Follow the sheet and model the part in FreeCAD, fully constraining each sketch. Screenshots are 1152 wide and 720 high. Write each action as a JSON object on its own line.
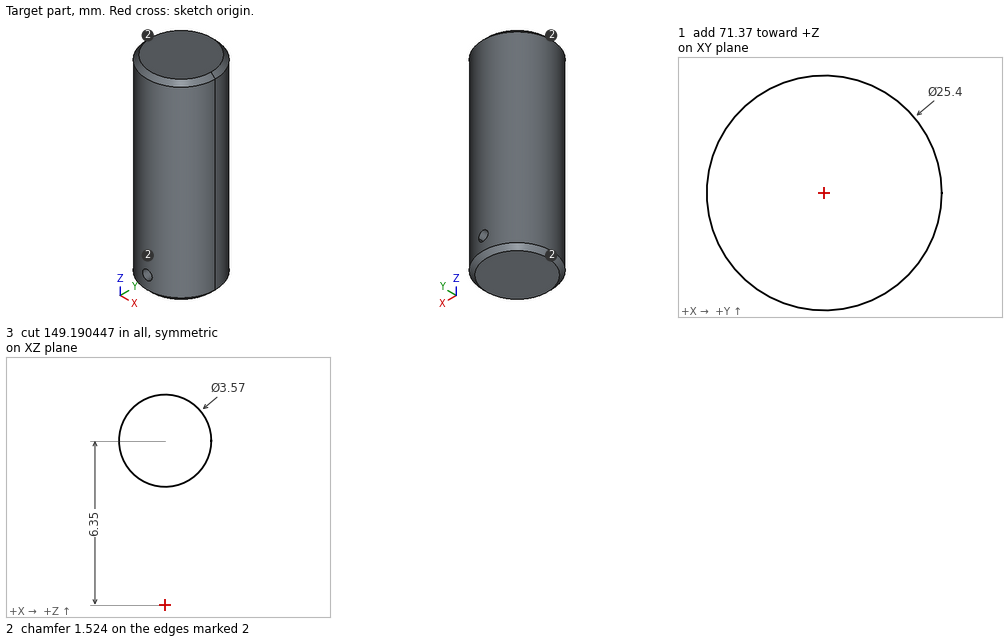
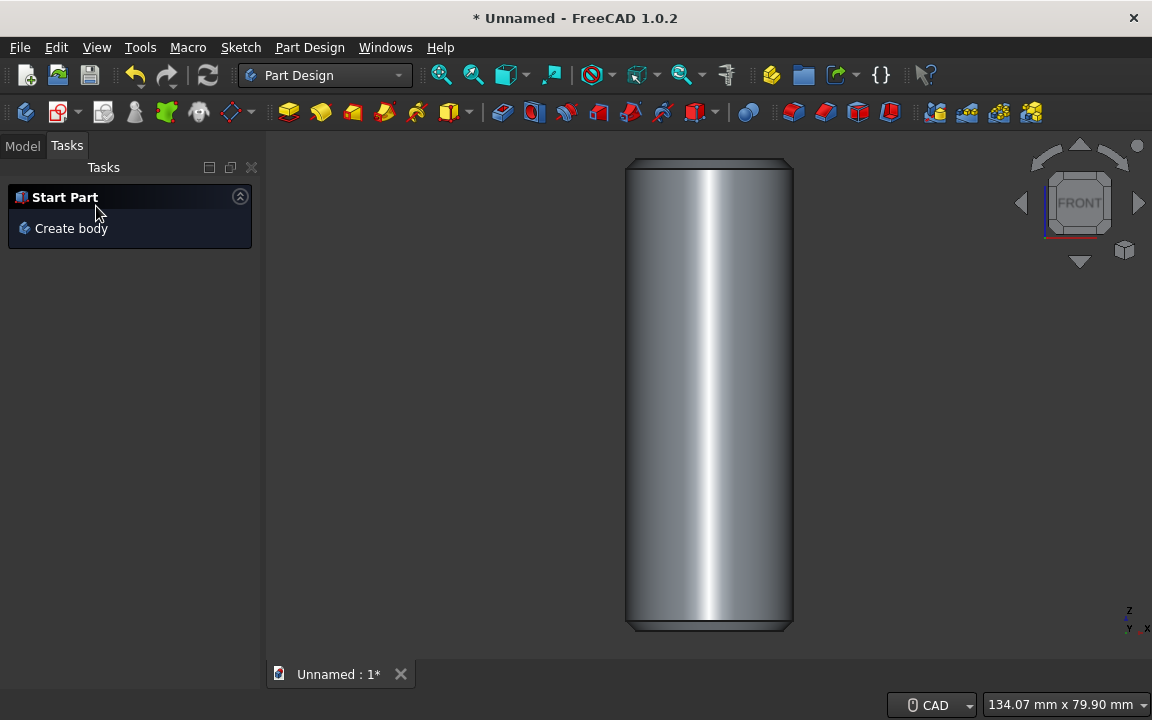
{"action": "left_click", "coordinate": [58, 112]}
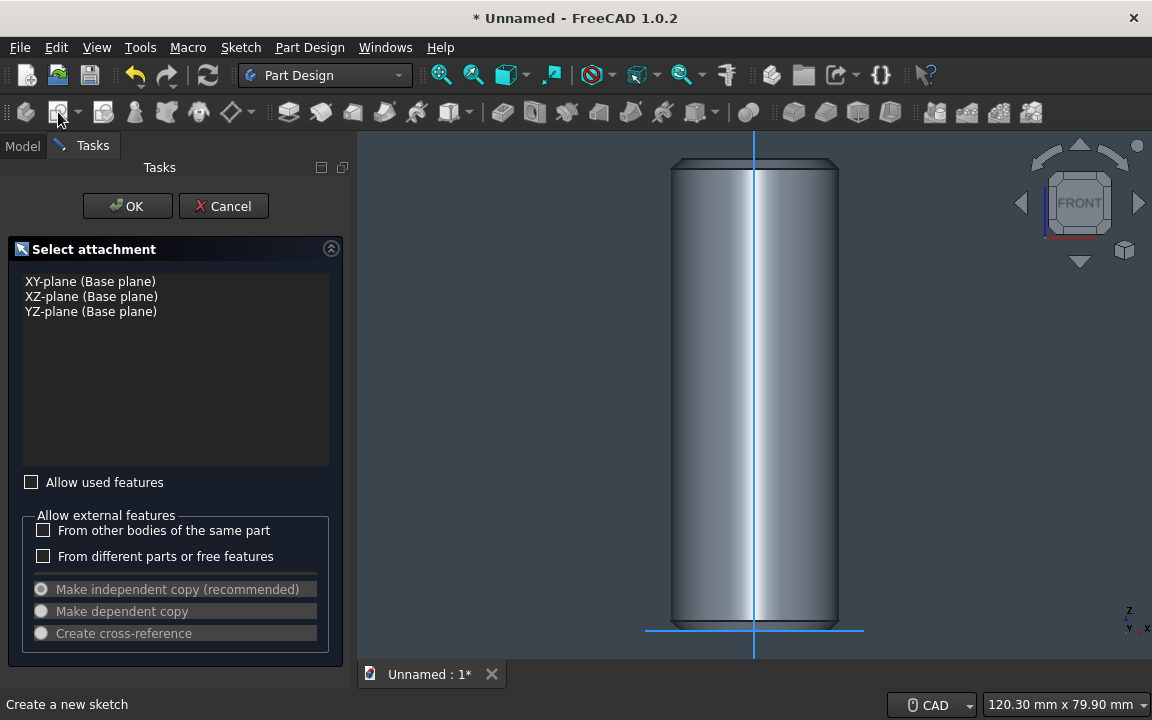
{"action": "left_click", "coordinate": [82, 296]}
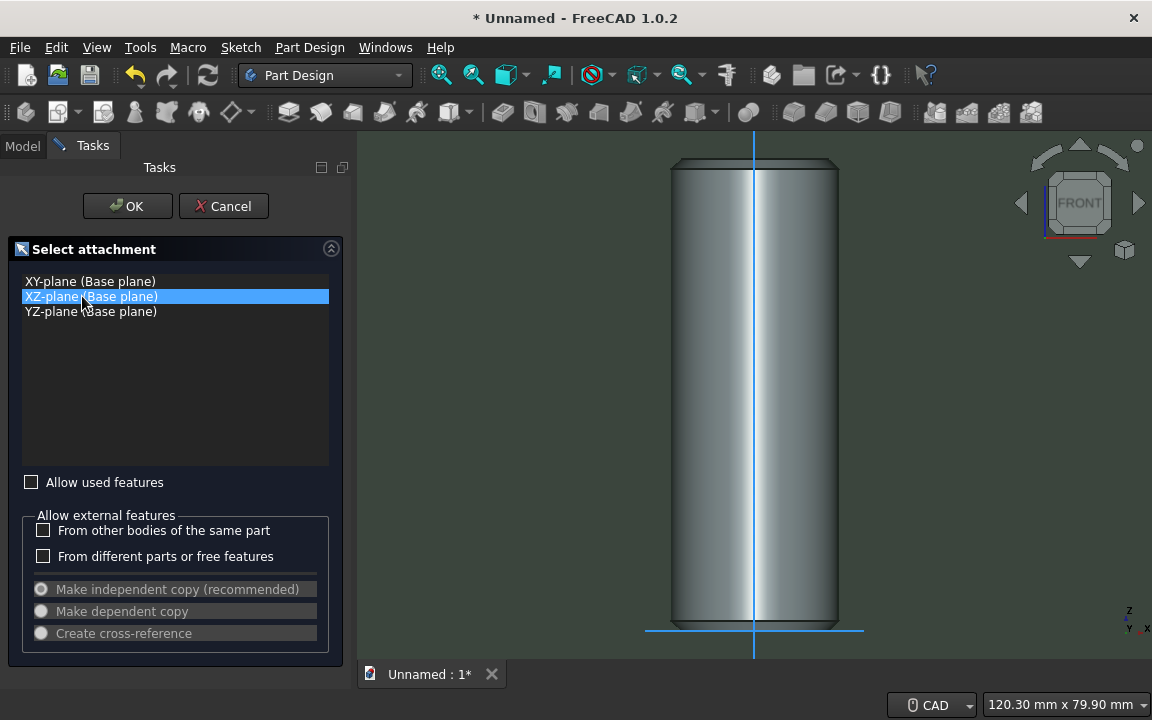
{"action": "left_click", "coordinate": [128, 206]}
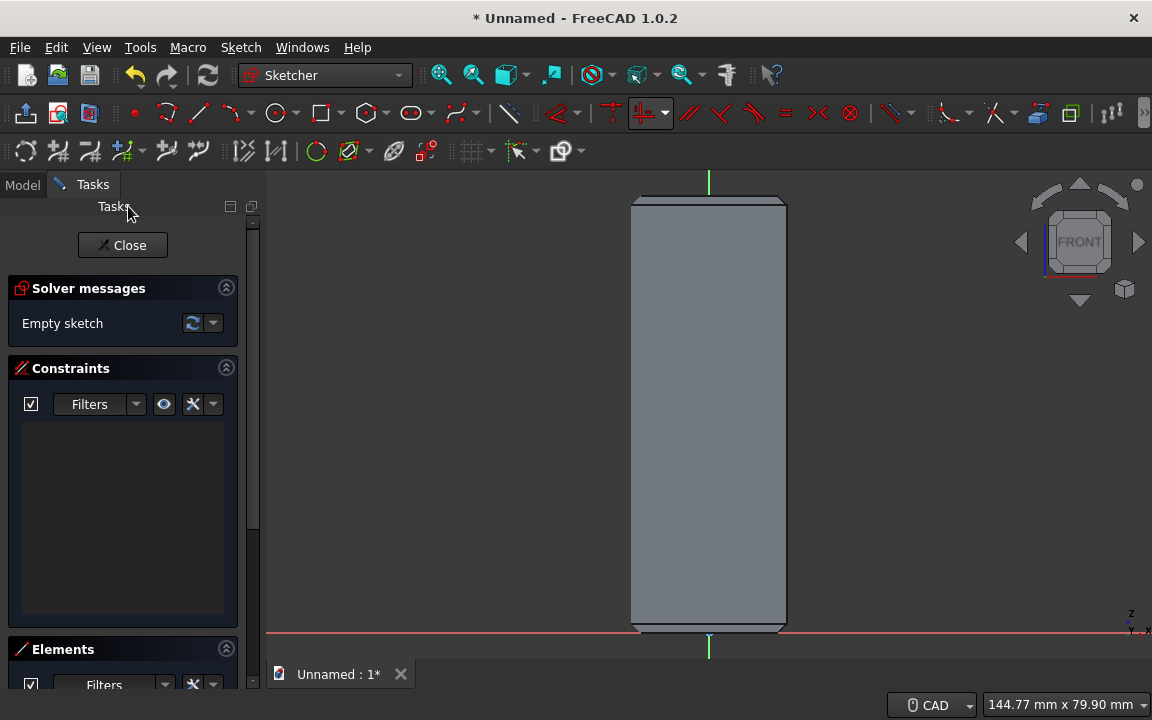
{"action": "left_click", "coordinate": [90, 114]}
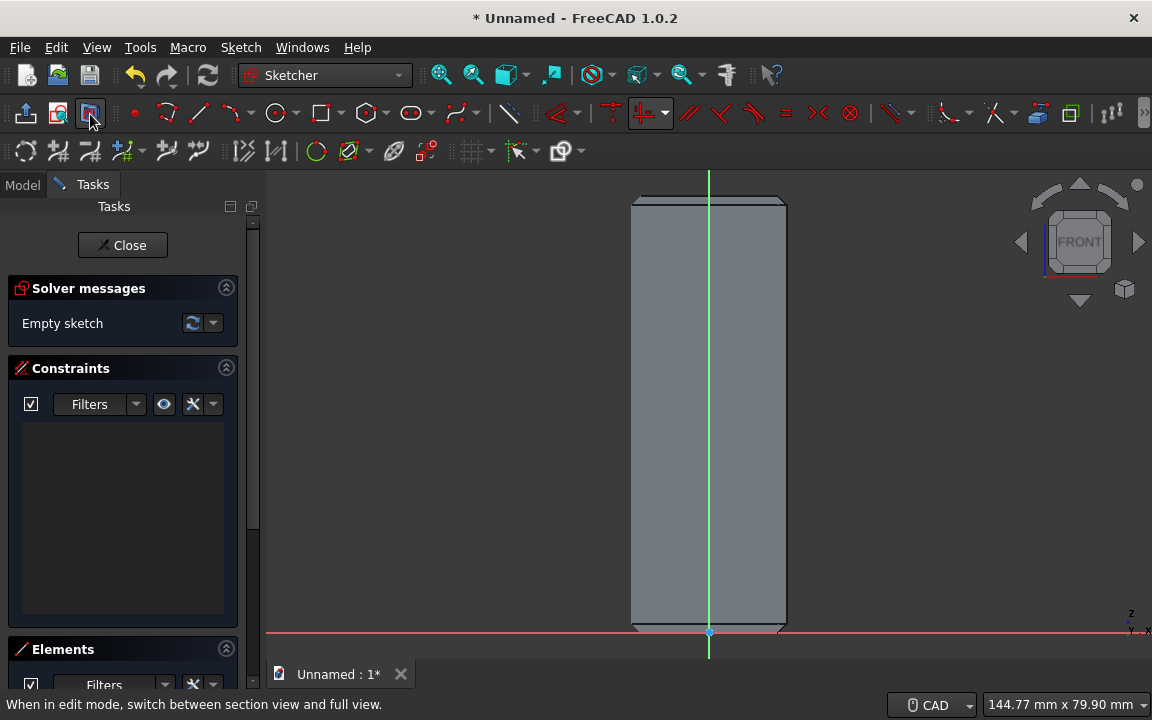
{"action": "scroll", "coordinate": [640, 414], "scroll_direction": "down", "scroll_amount": 5}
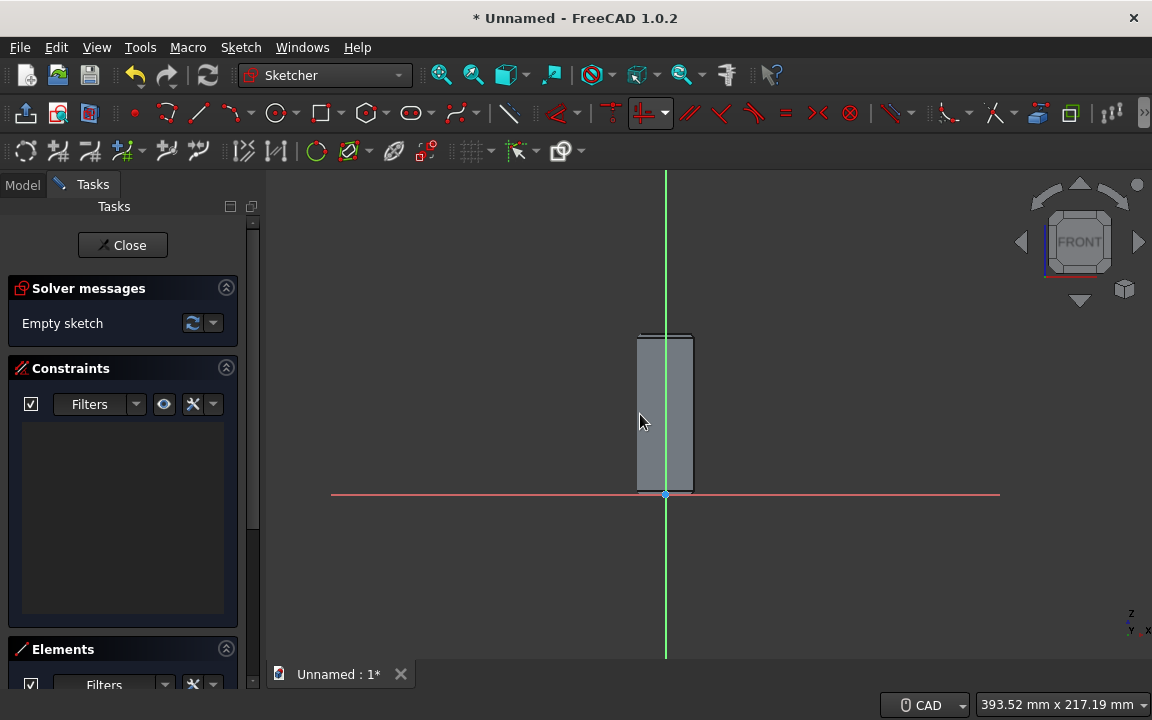
{"action": "scroll", "coordinate": [667, 490], "scroll_direction": "up", "scroll_amount": 14}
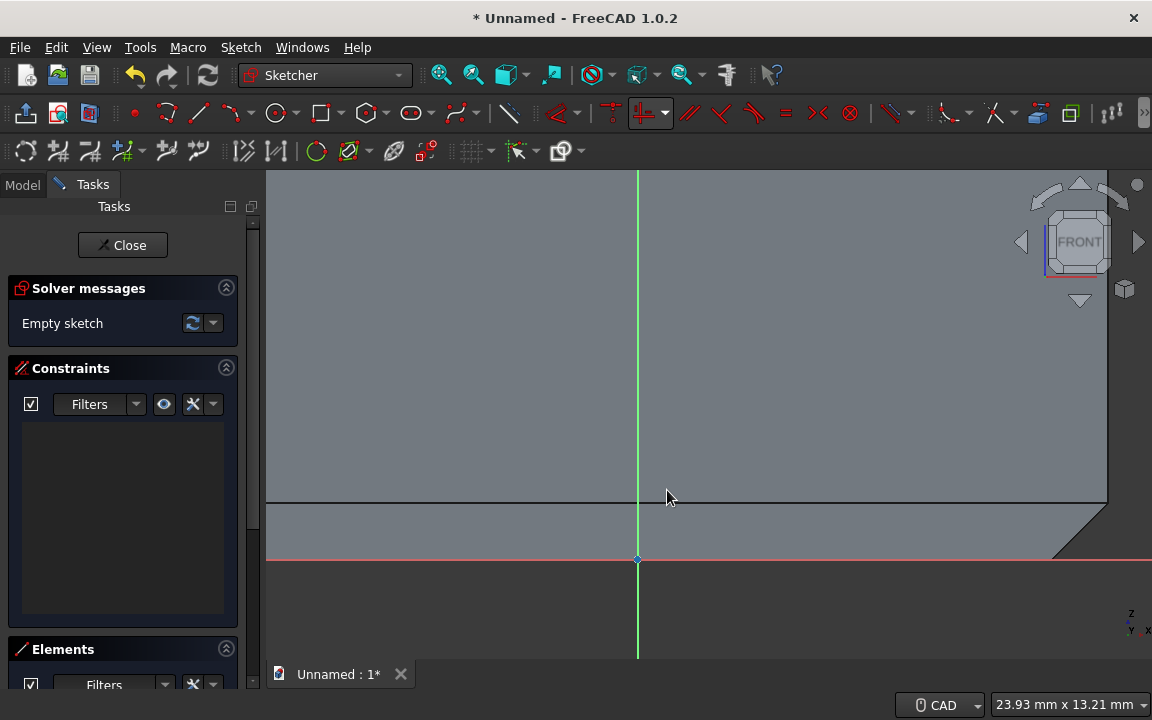
{"action": "left_click", "coordinate": [276, 114]}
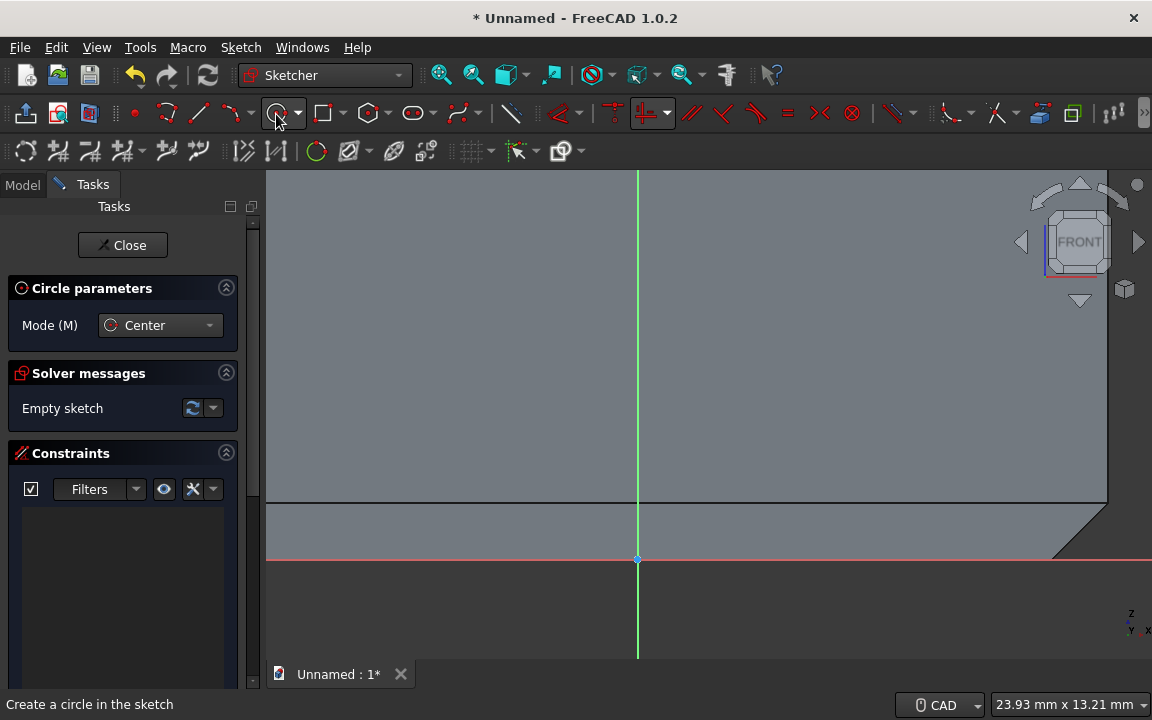
{"action": "left_click", "coordinate": [638, 324]}
{"action": "left_click", "coordinate": [685, 278]}
{"action": "key", "text": "Escape"}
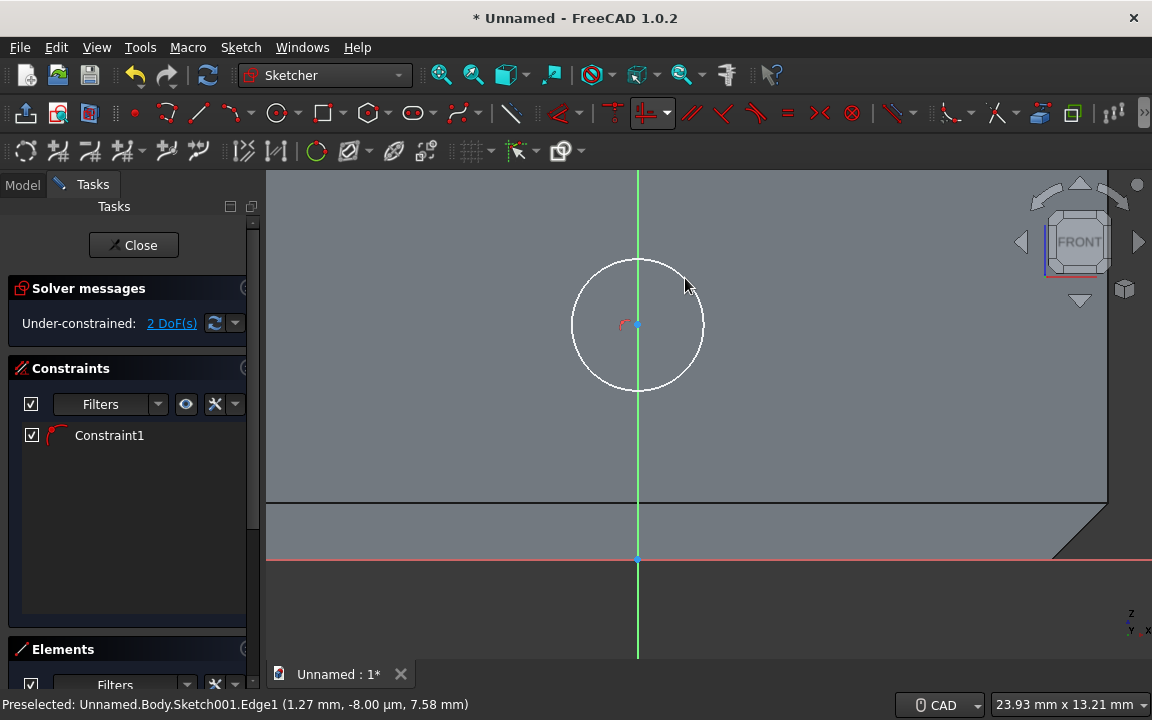
{"action": "left_click", "coordinate": [558, 114]}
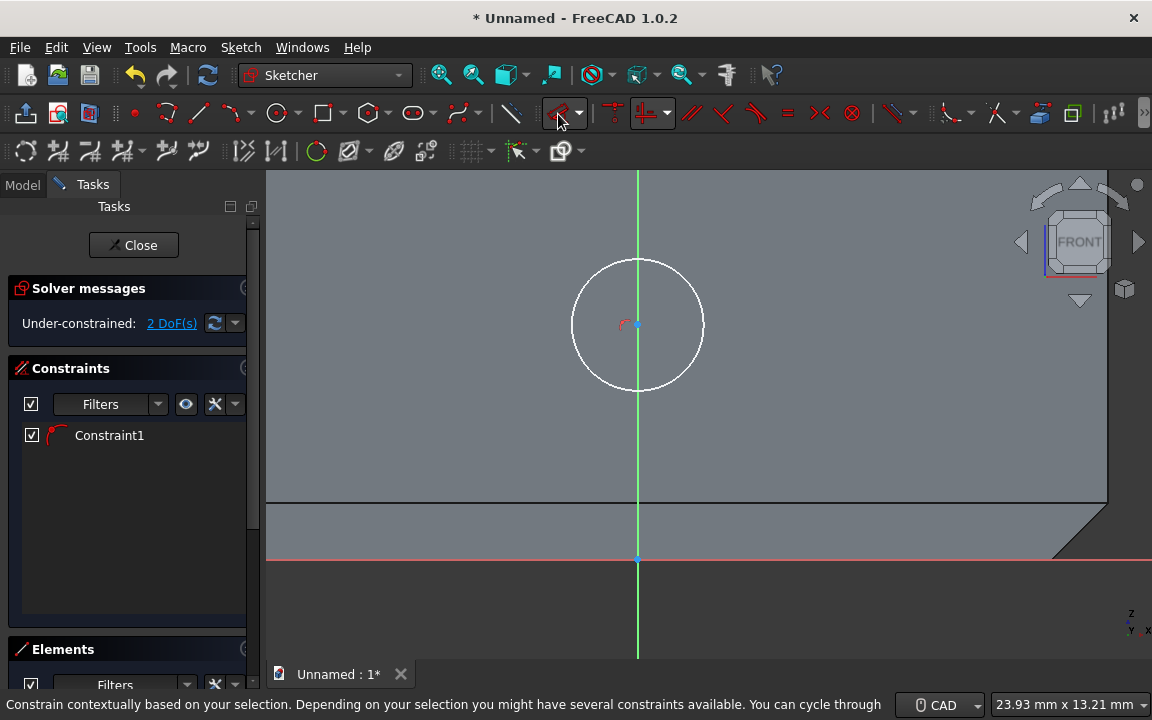
{"action": "left_click", "coordinate": [684, 278]}
{"action": "left_click", "coordinate": [706, 255]}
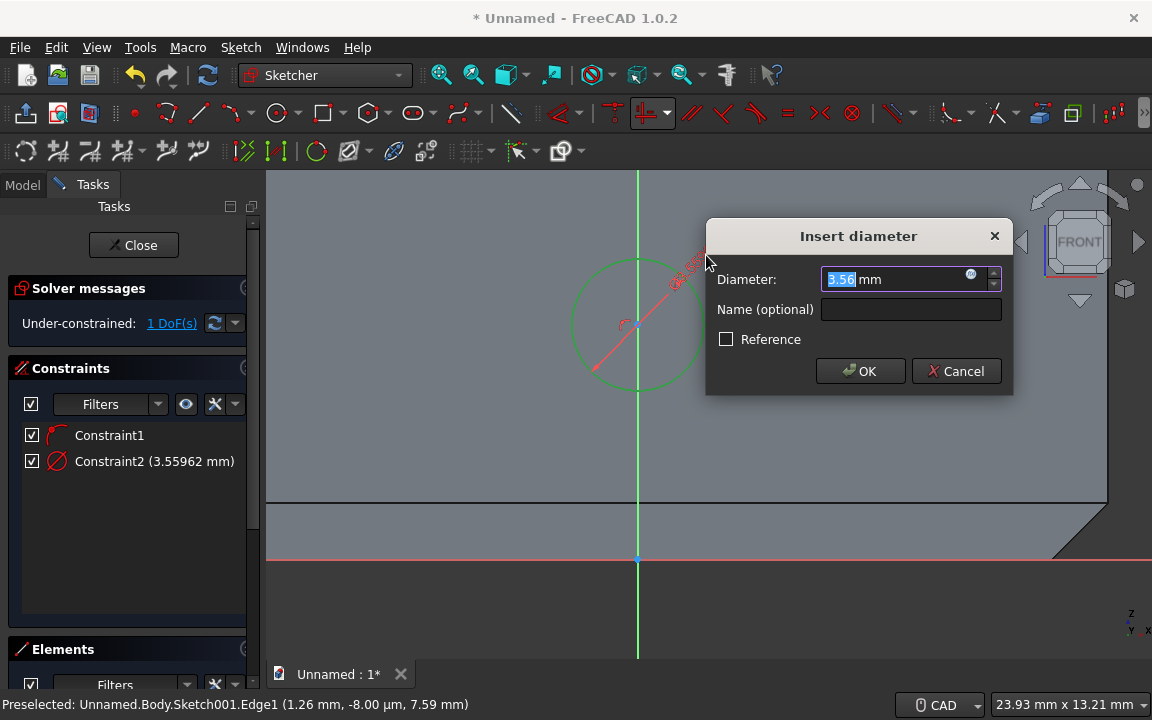
{"action": "type", "text": "3.57"}
{"action": "key", "text": "Return"}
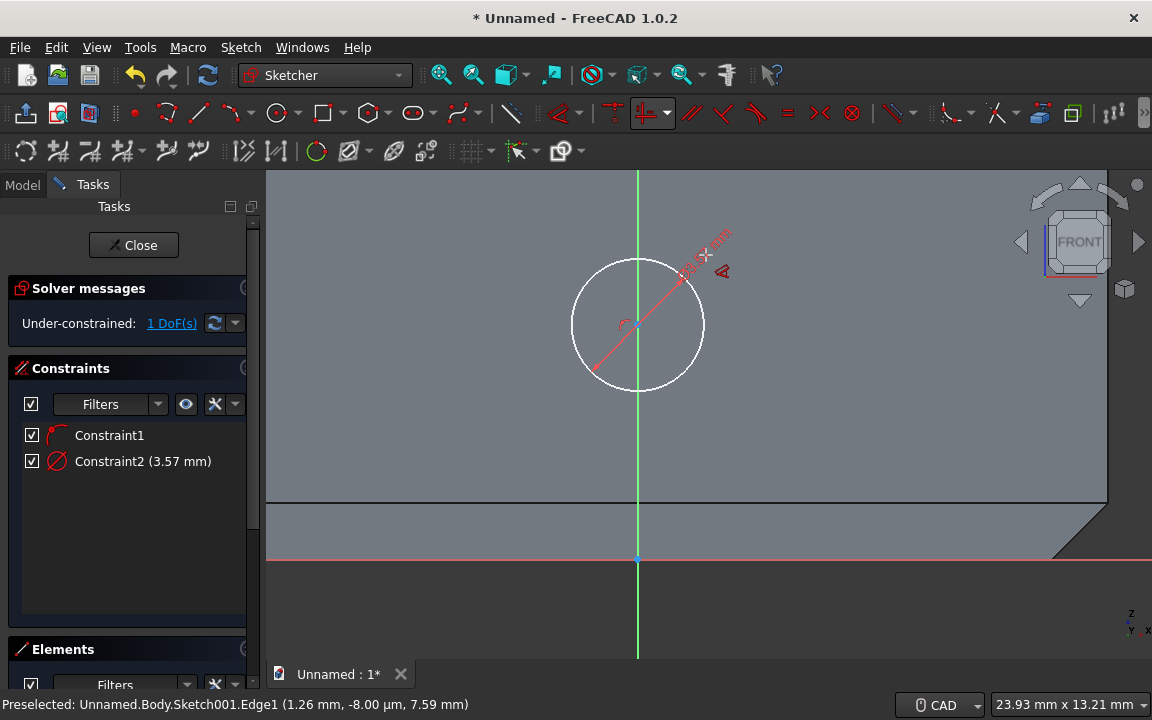
{"action": "left_click", "coordinate": [638, 325]}
{"action": "left_click", "coordinate": [672, 442]}